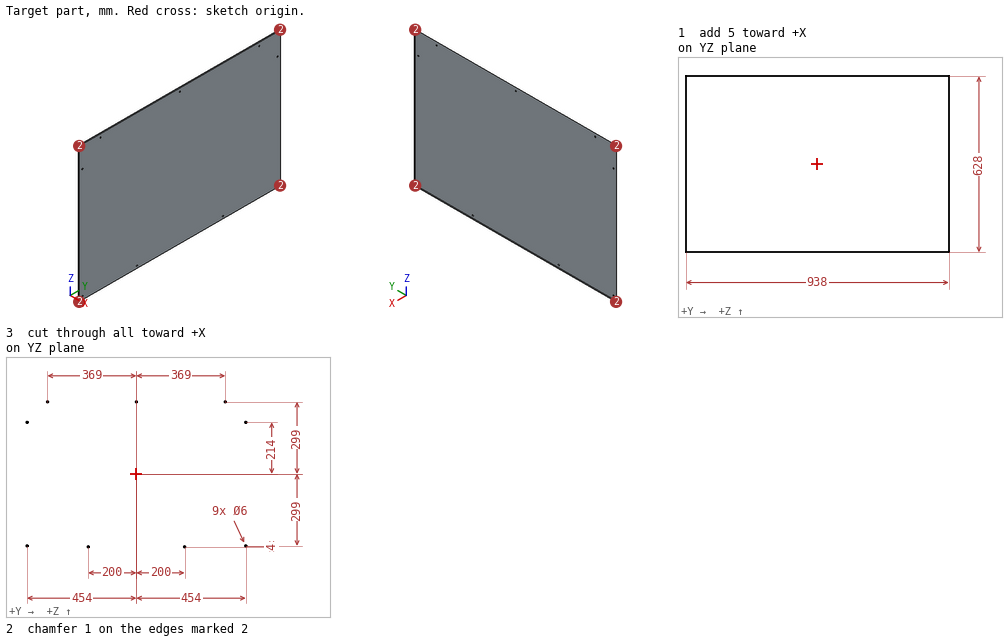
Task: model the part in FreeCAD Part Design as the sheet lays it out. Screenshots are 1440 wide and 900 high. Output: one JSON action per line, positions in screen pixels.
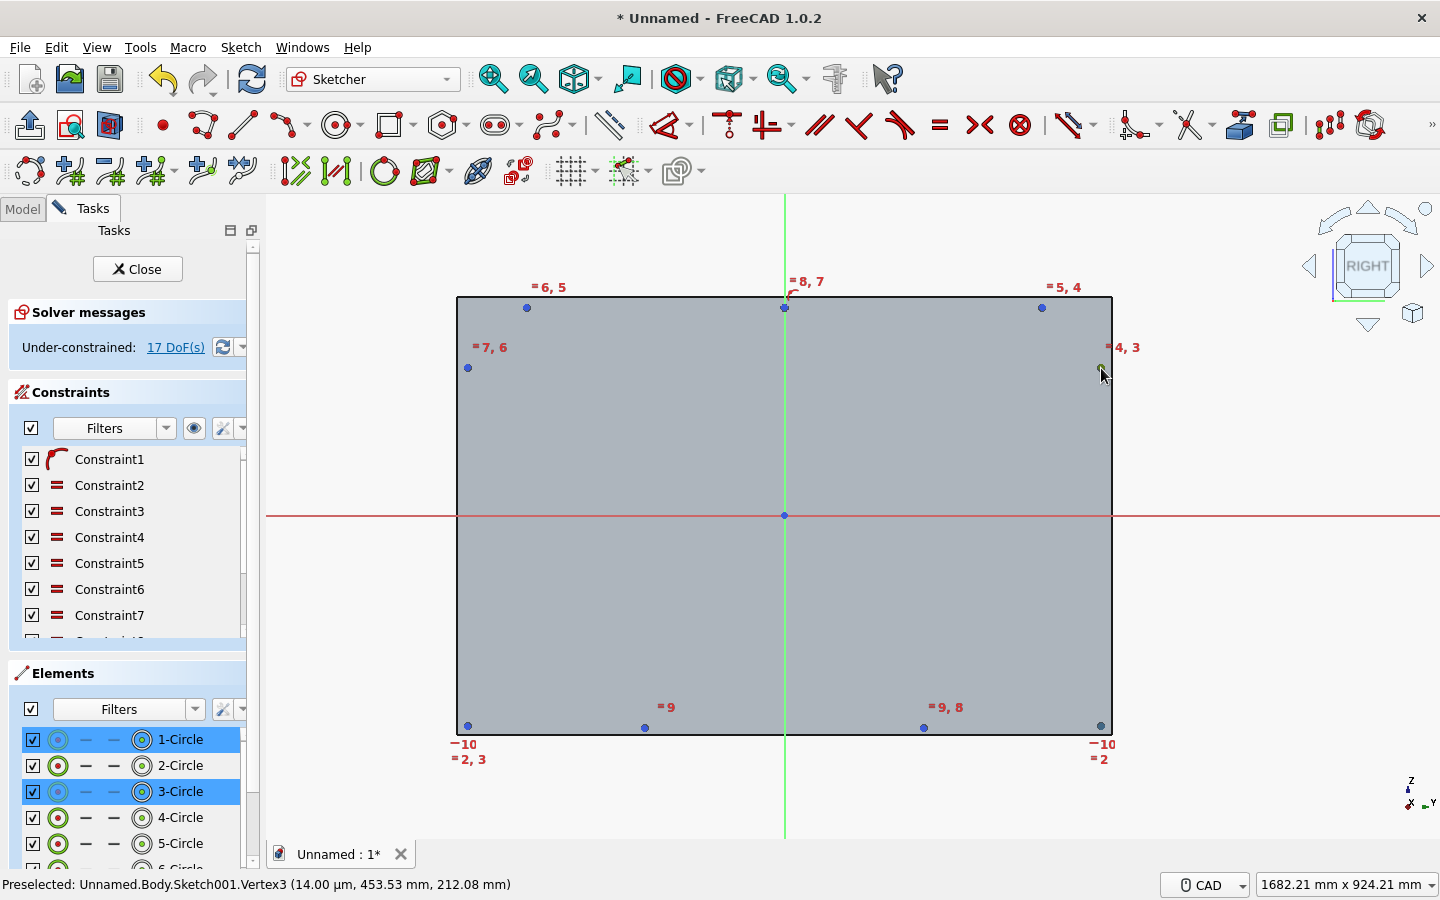
{"action": "key", "text": "v"}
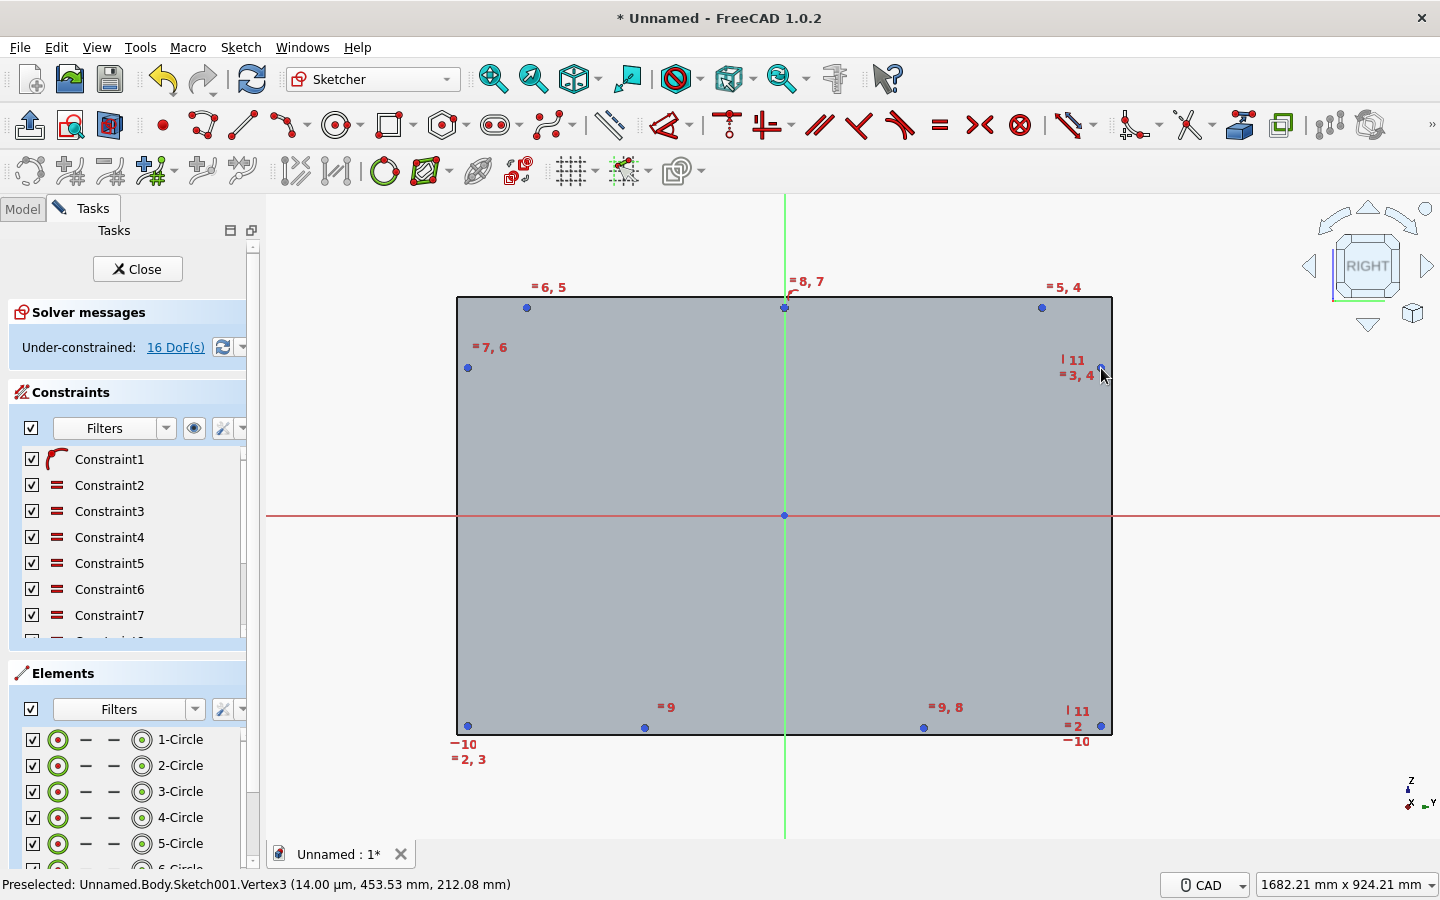
{"action": "left_click", "coordinate": [1042, 308]}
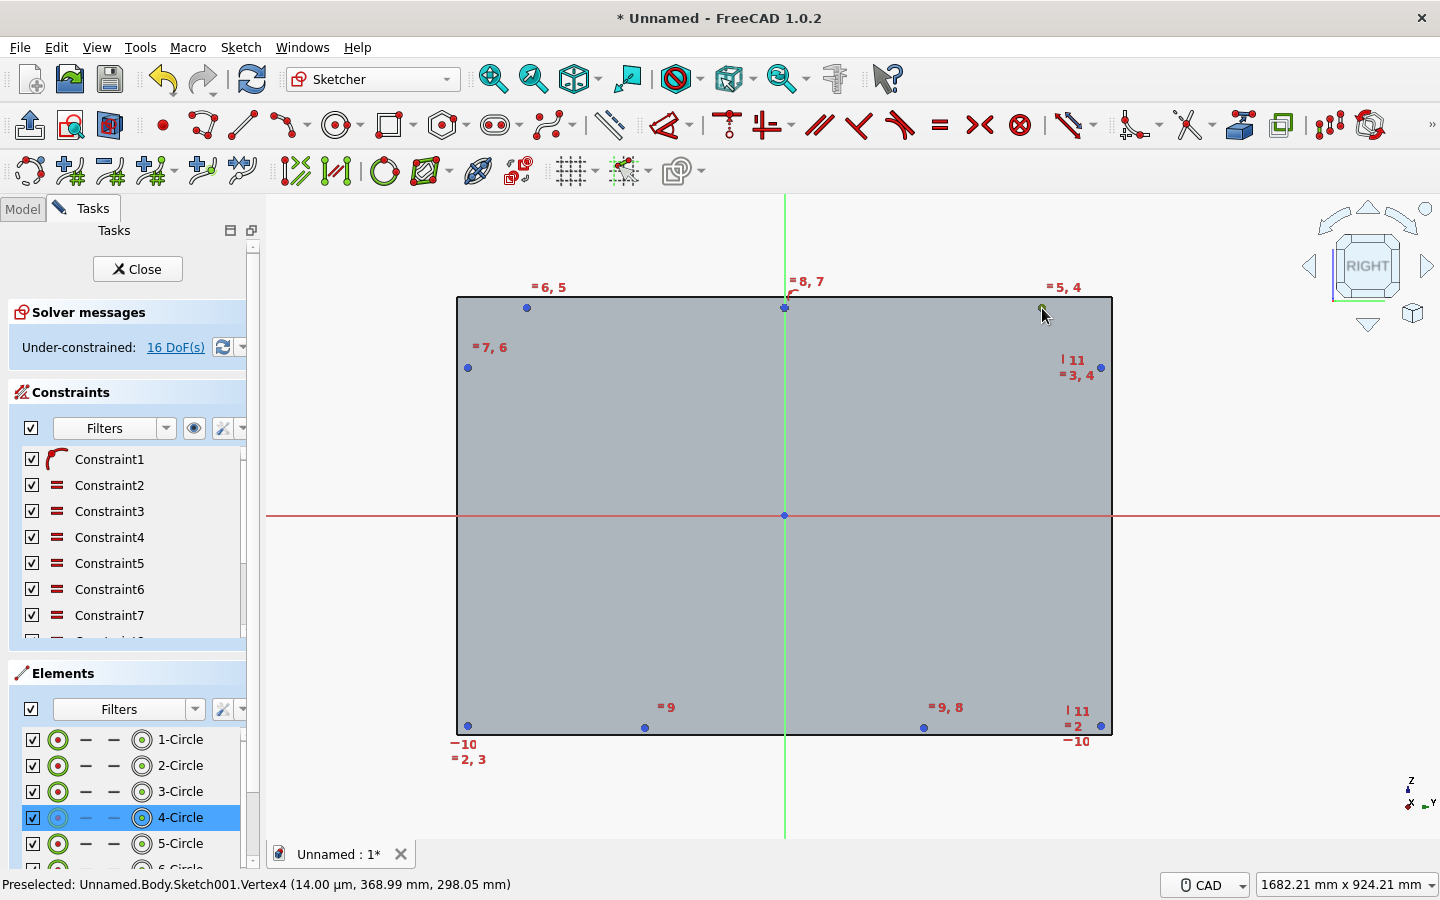
{"action": "left_click", "coordinate": [527, 308]}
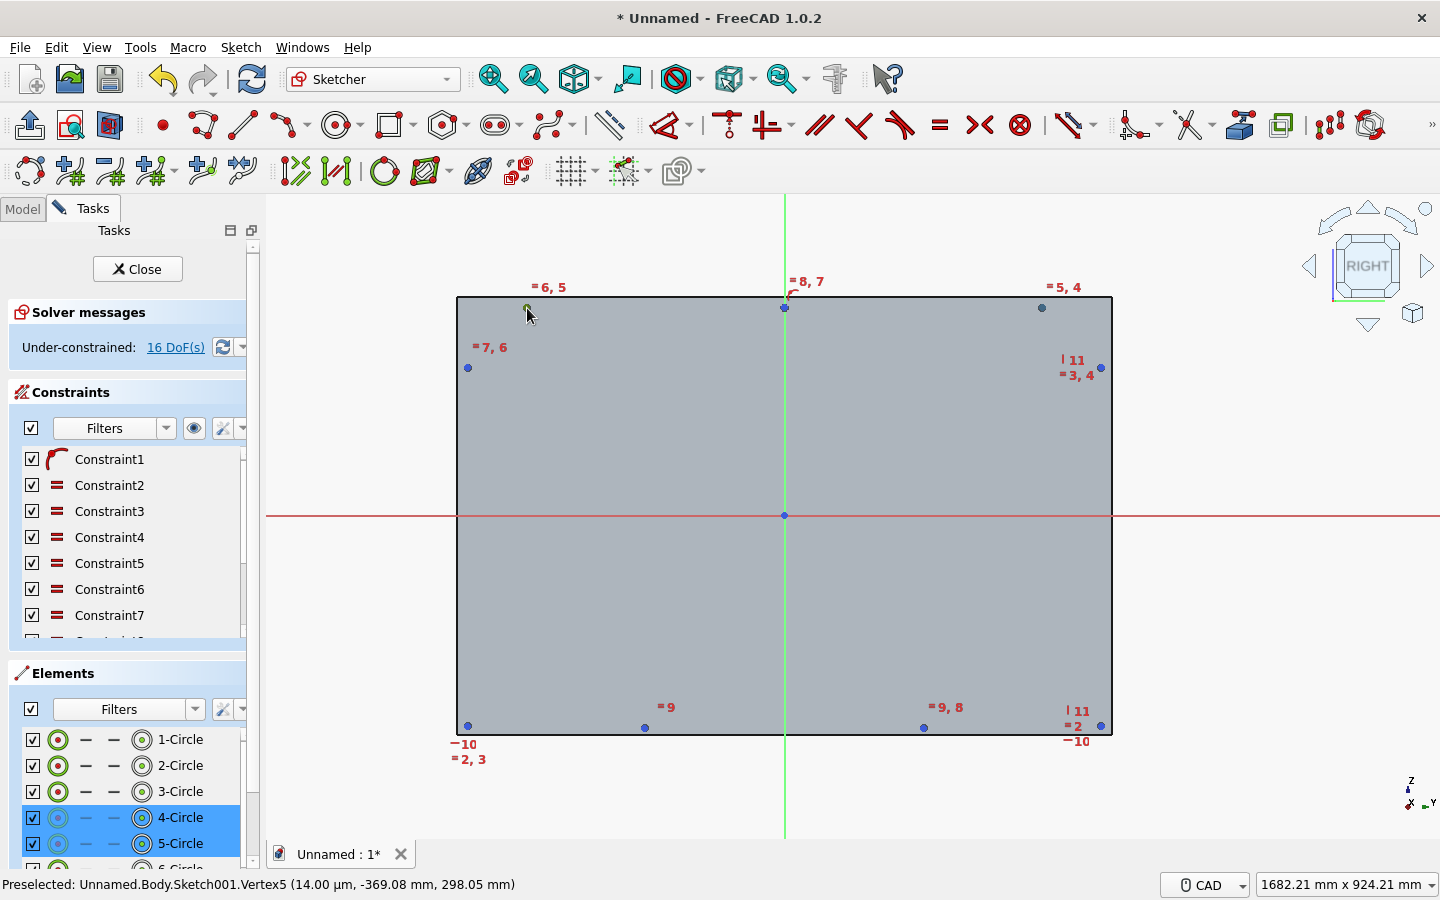
{"action": "key", "text": "h"}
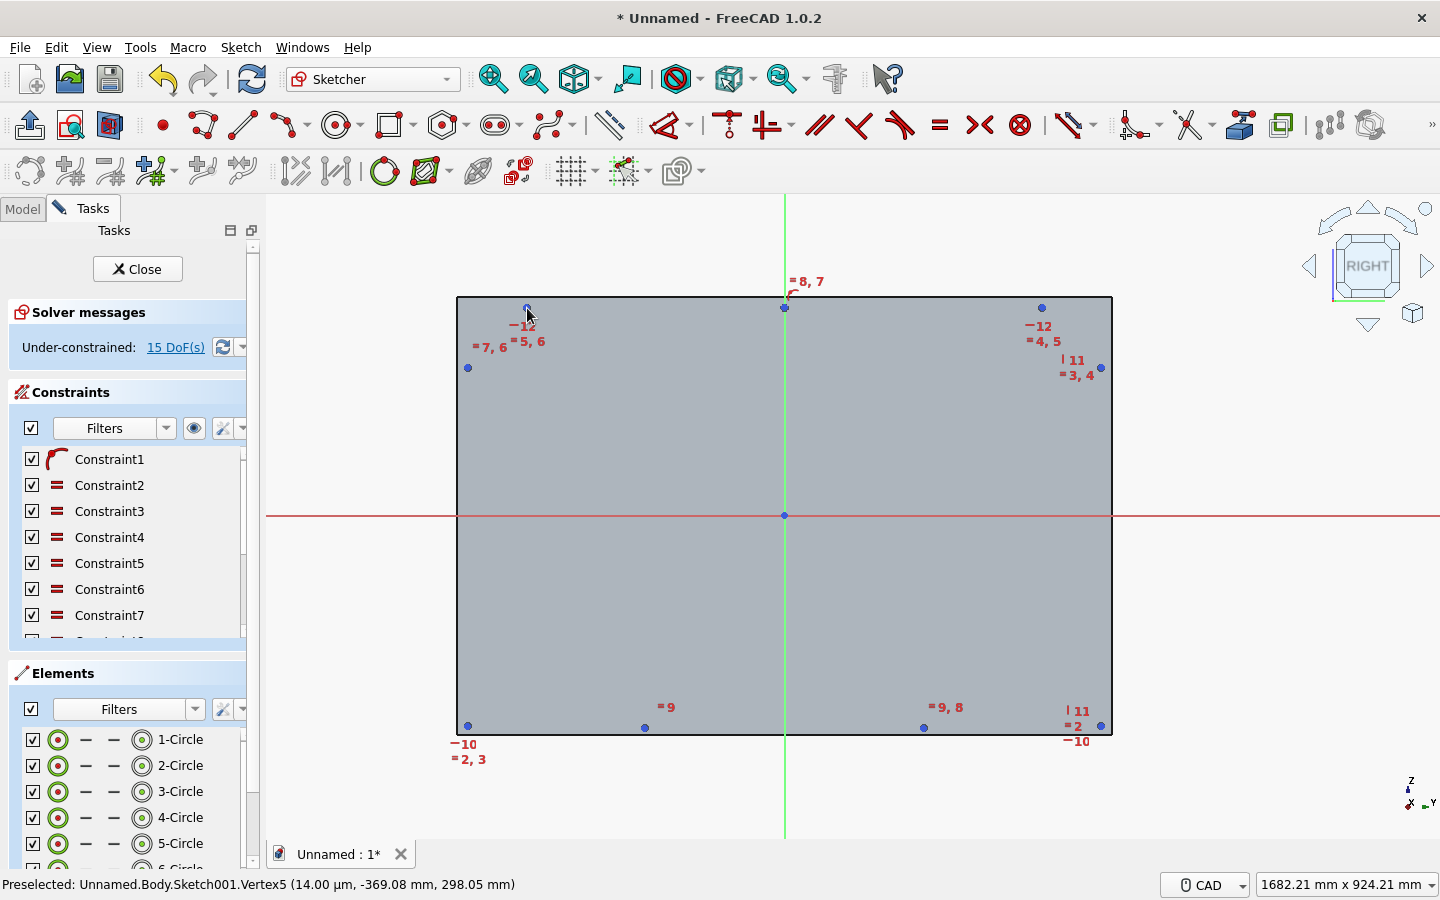
{"action": "left_click", "coordinate": [468, 726]}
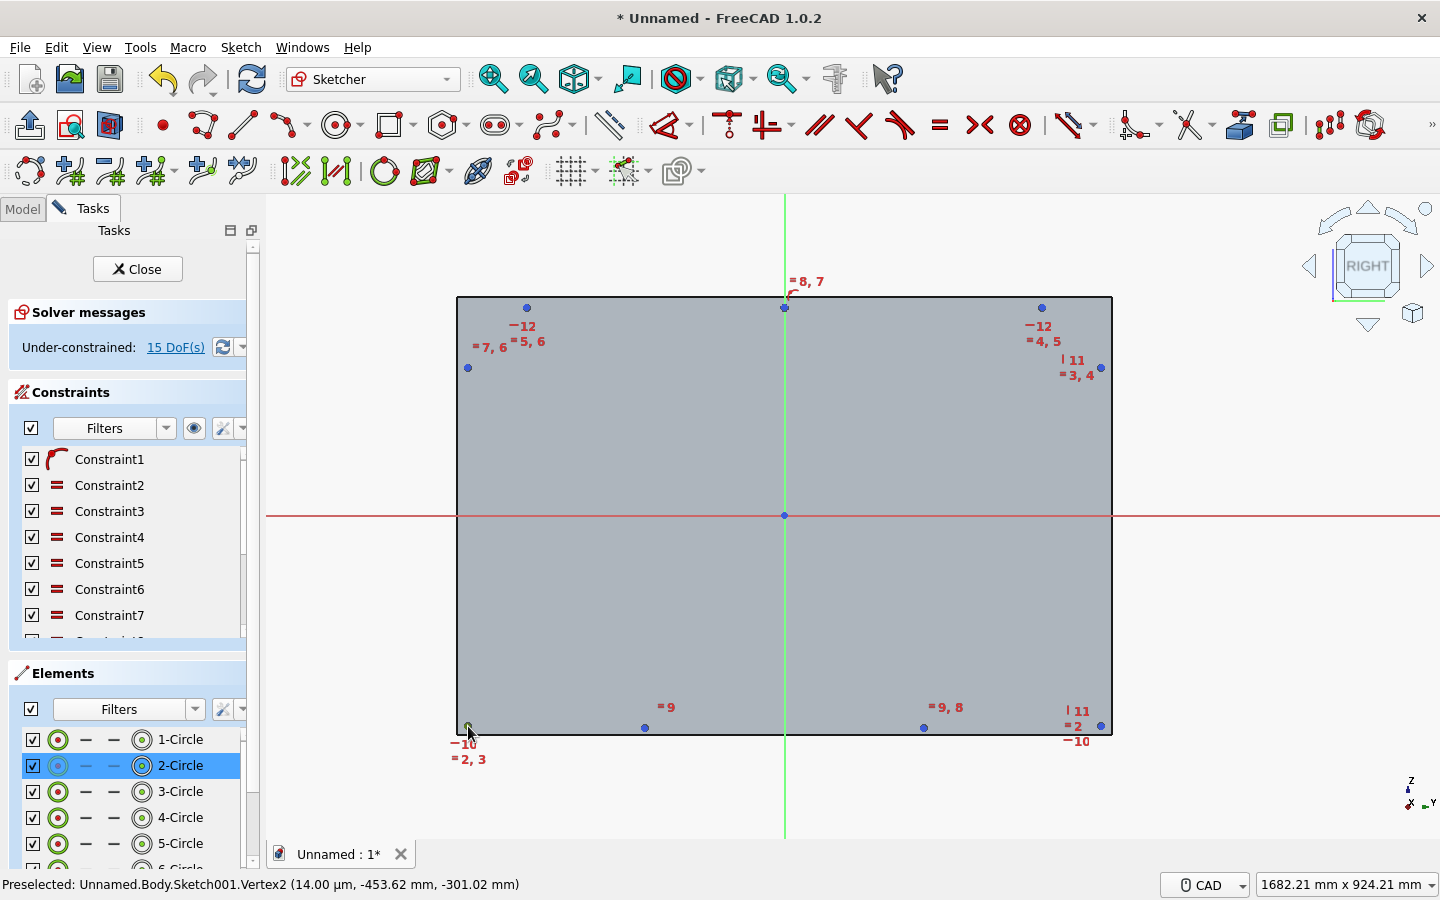
{"action": "left_click", "coordinate": [468, 368]}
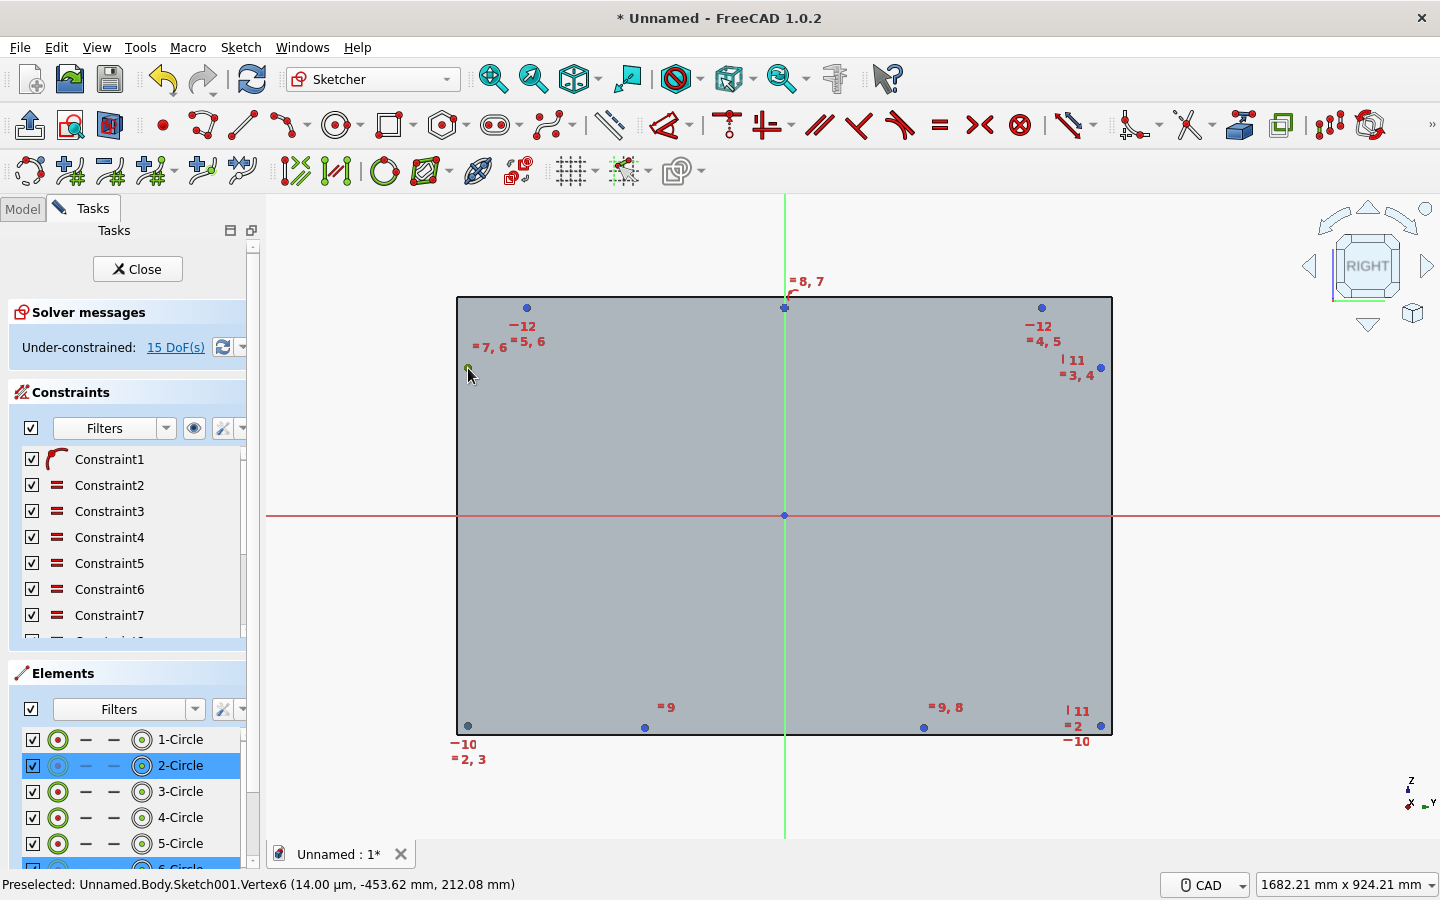
{"action": "key", "text": "v"}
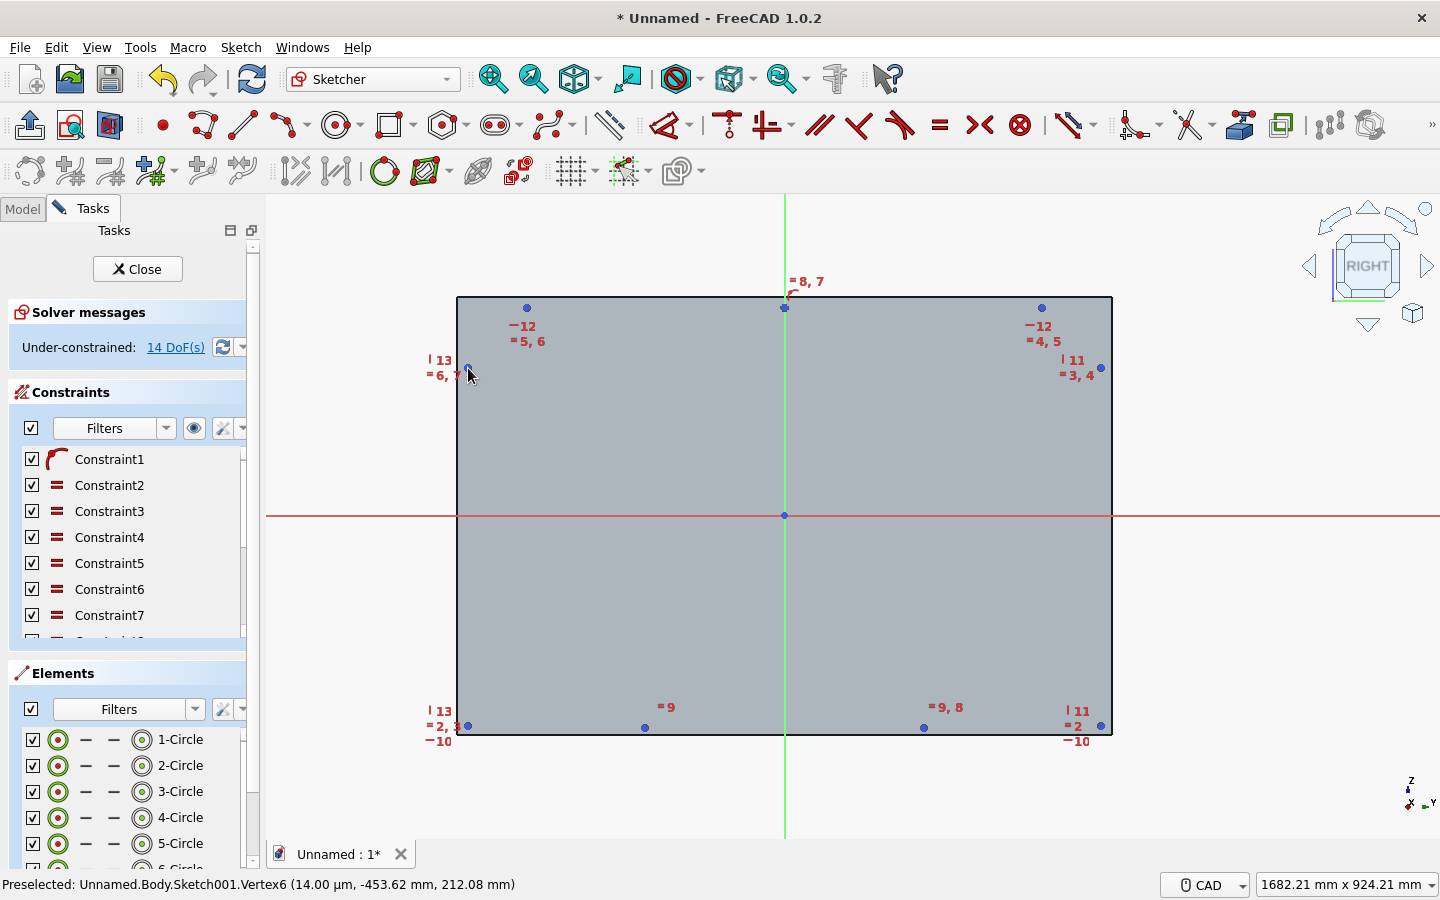
{"action": "left_click", "coordinate": [1101, 368]}